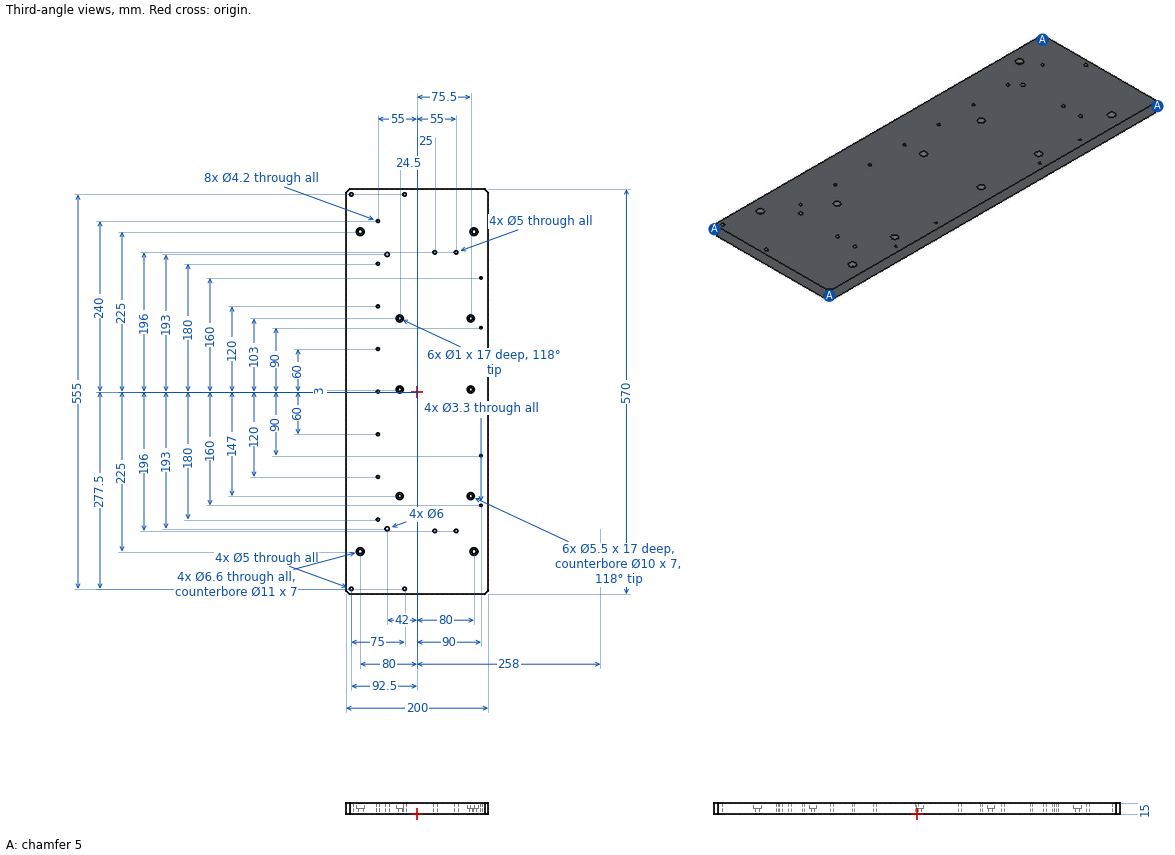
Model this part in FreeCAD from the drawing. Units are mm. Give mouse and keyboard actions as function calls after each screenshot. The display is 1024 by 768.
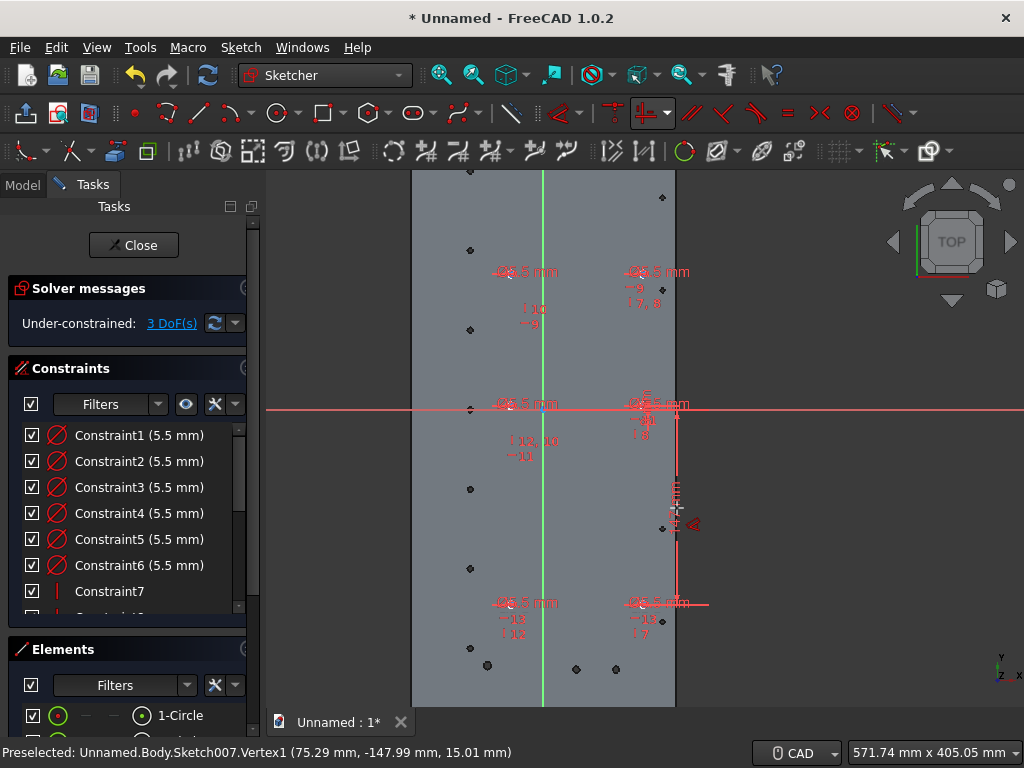
click(643, 274)
click(677, 342)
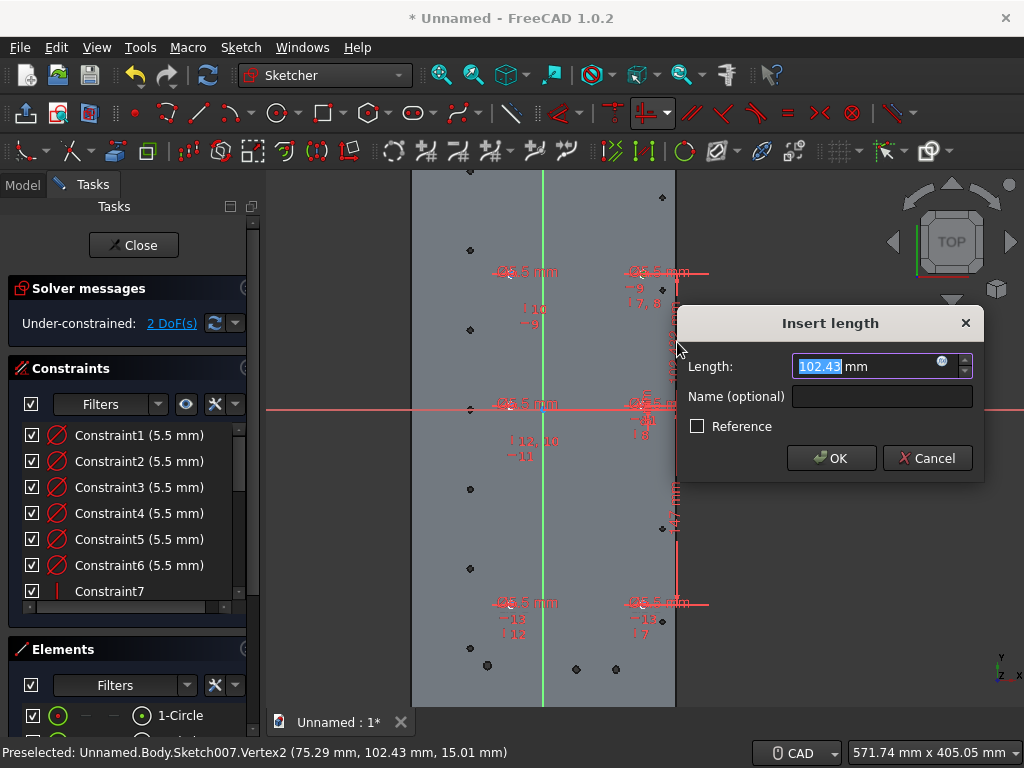
text(103)
key(Return)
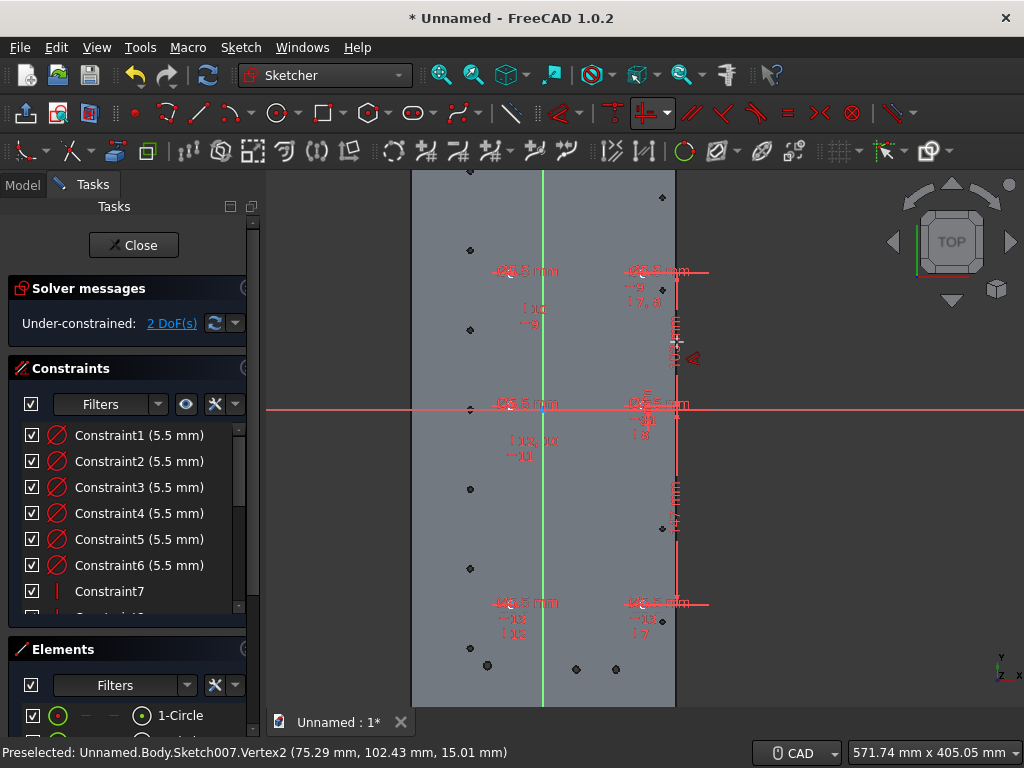
click(643, 605)
click(593, 639)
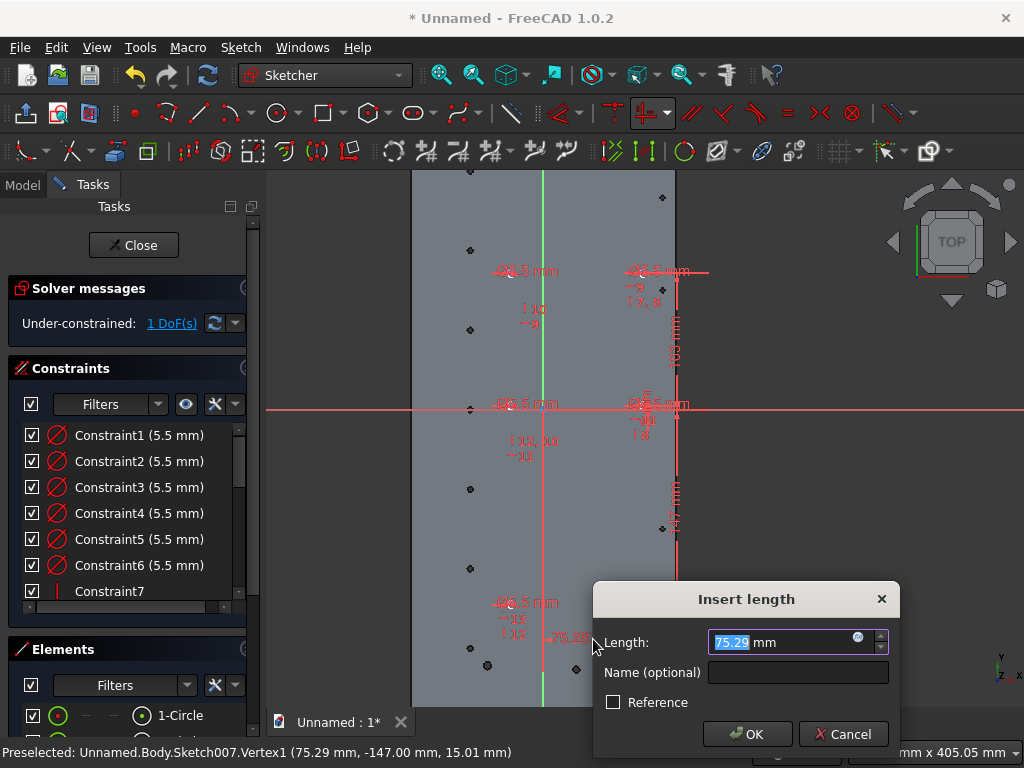
text(75.5)
key(Return)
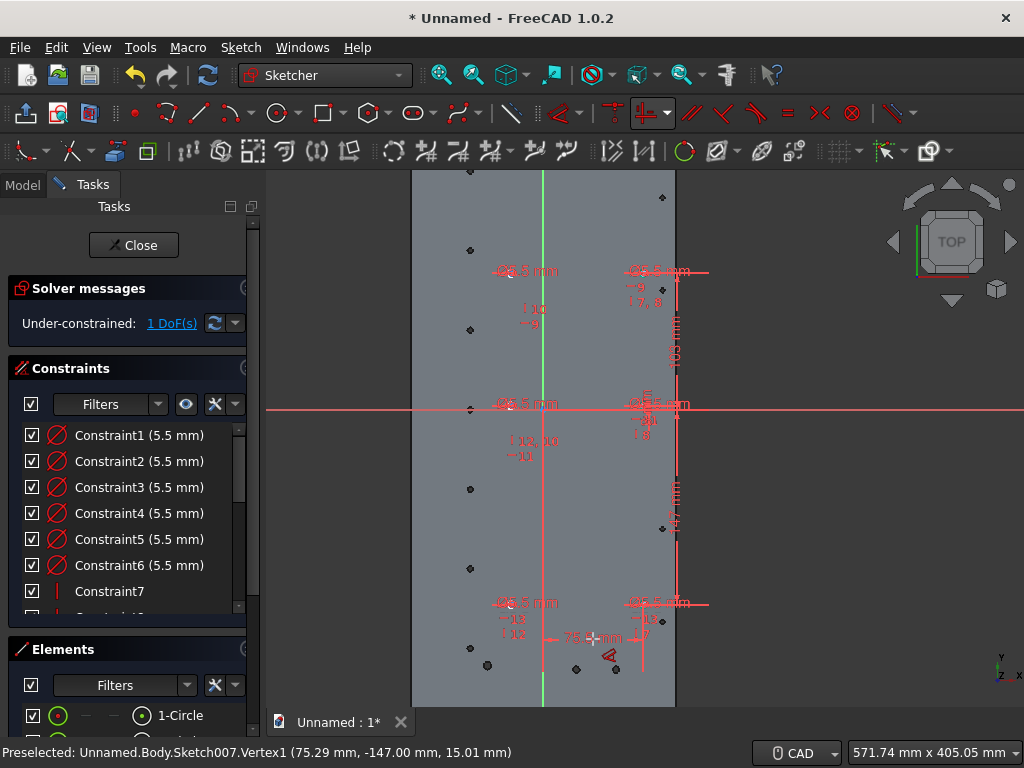
scroll(511, 273, up, 2)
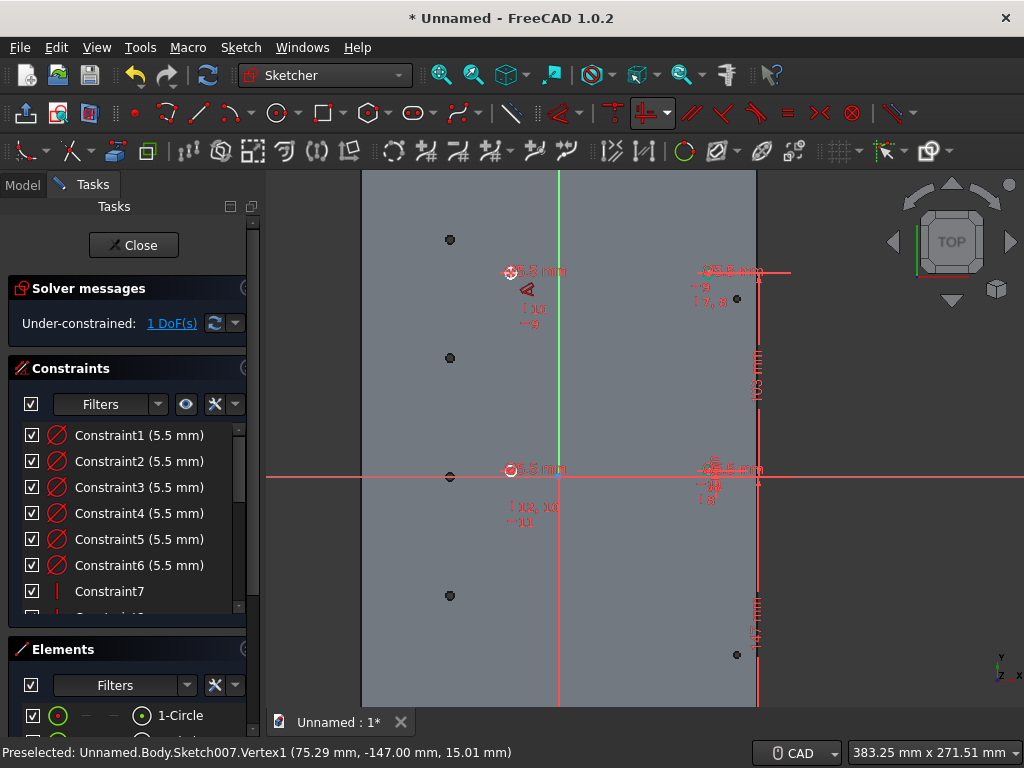
click(511, 273)
click(535, 239)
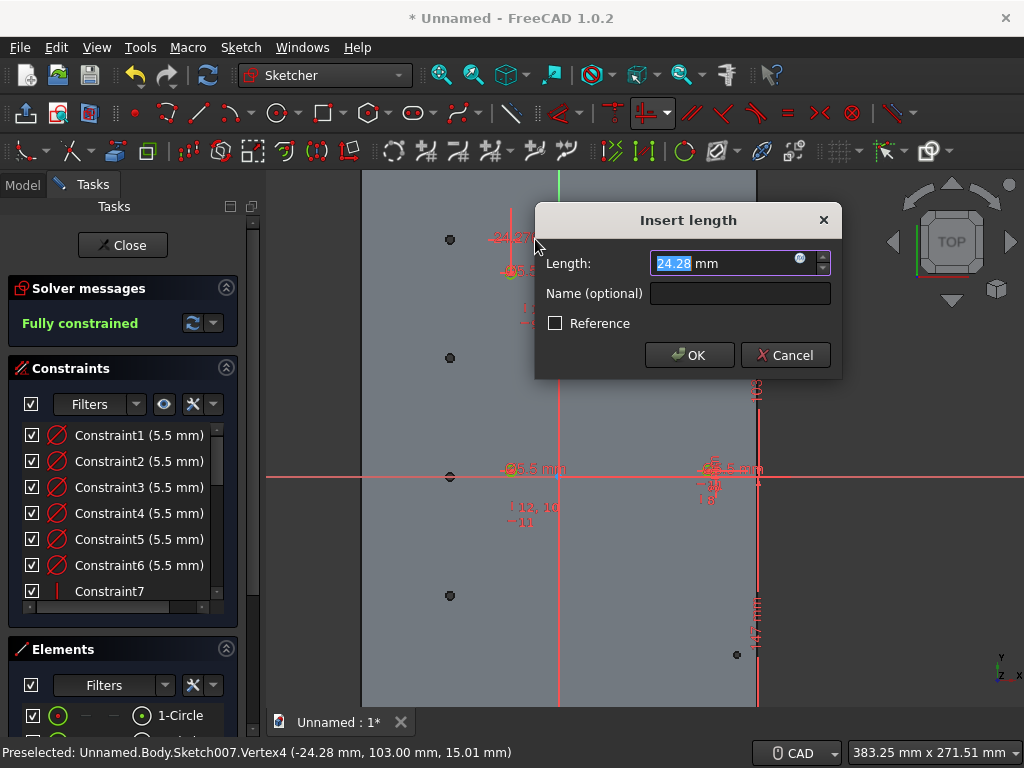
text(24.5)
key(Return)
key(Escape)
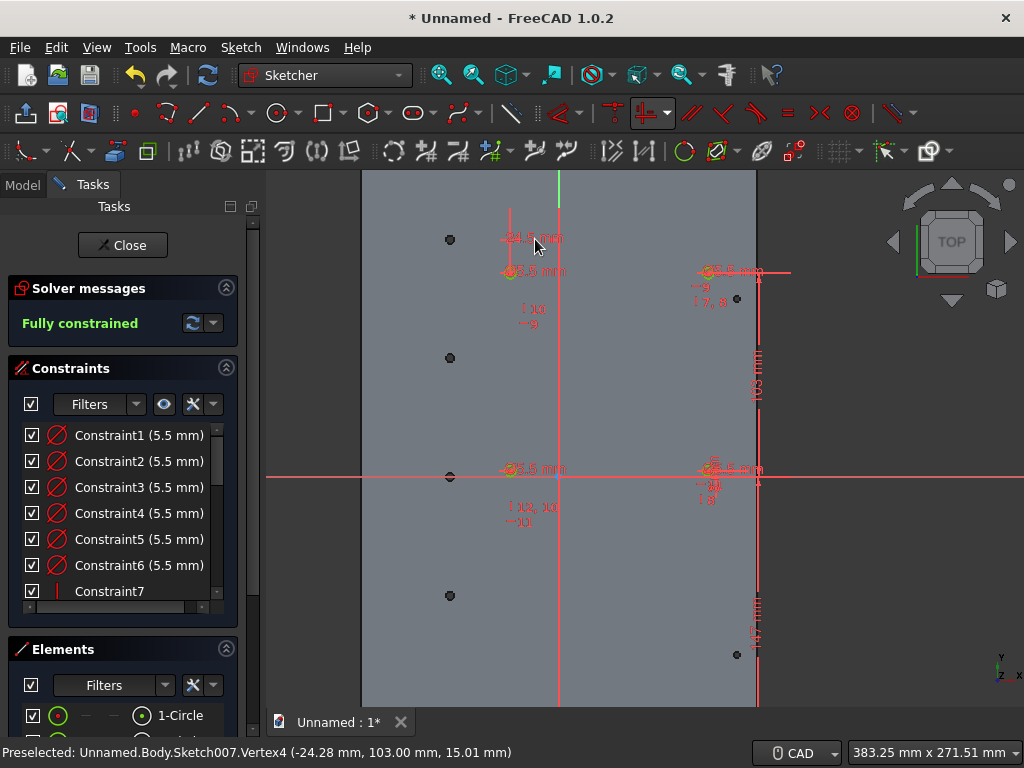
click(123, 245)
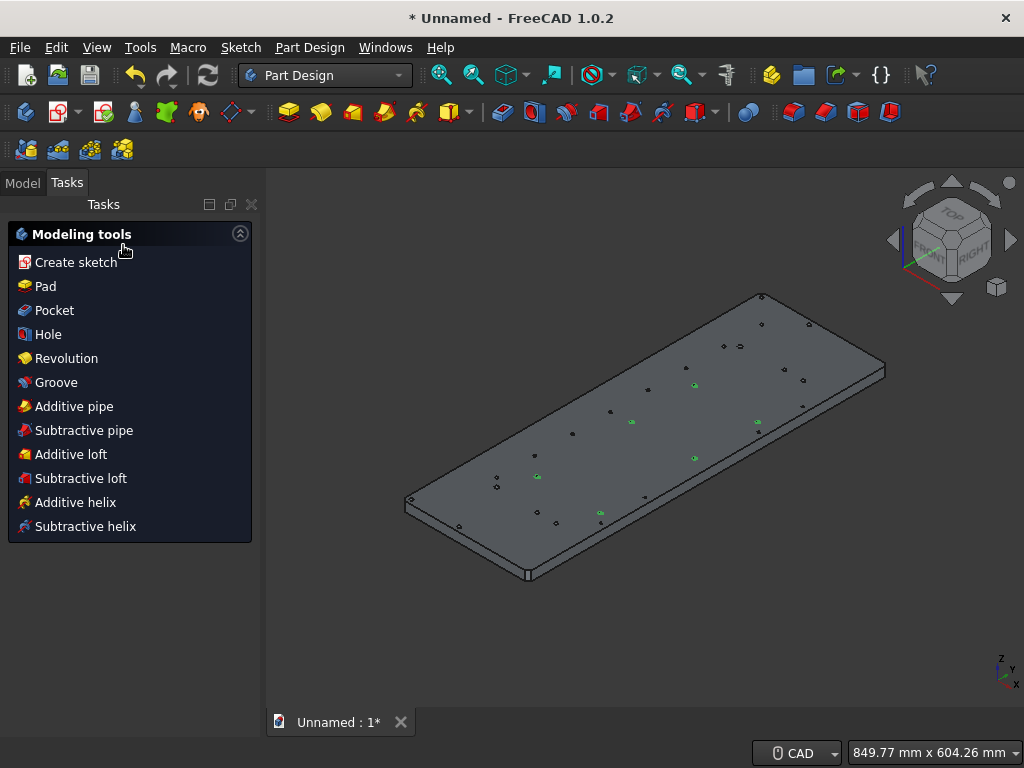
click(536, 112)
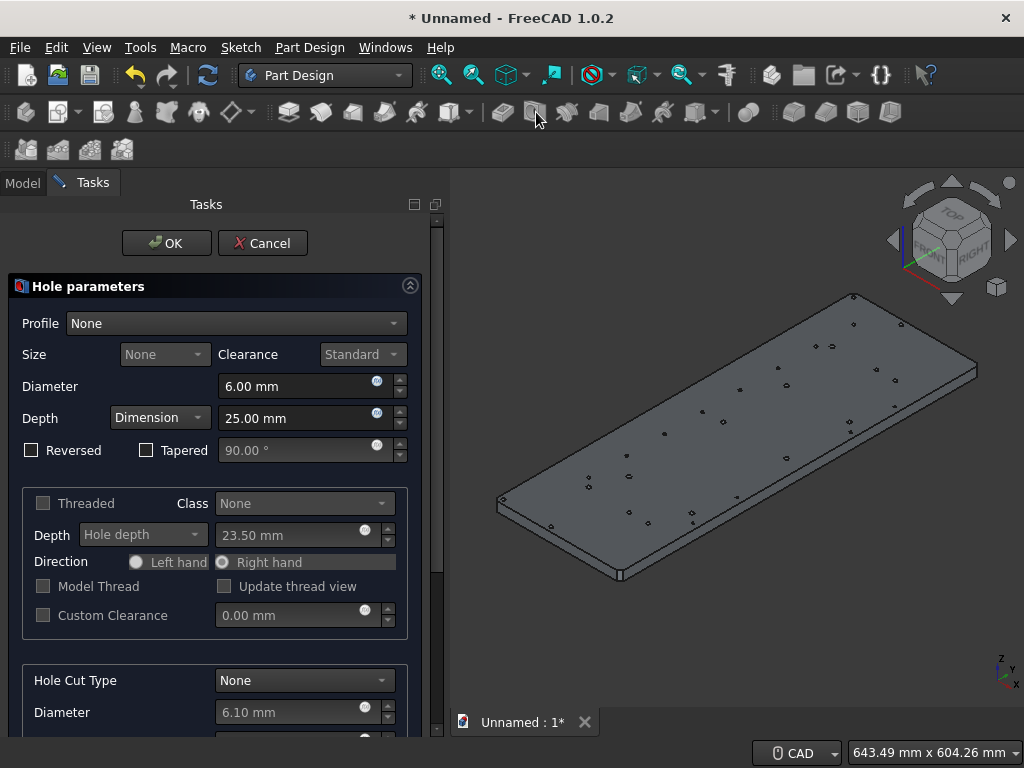
triple_click(305, 386)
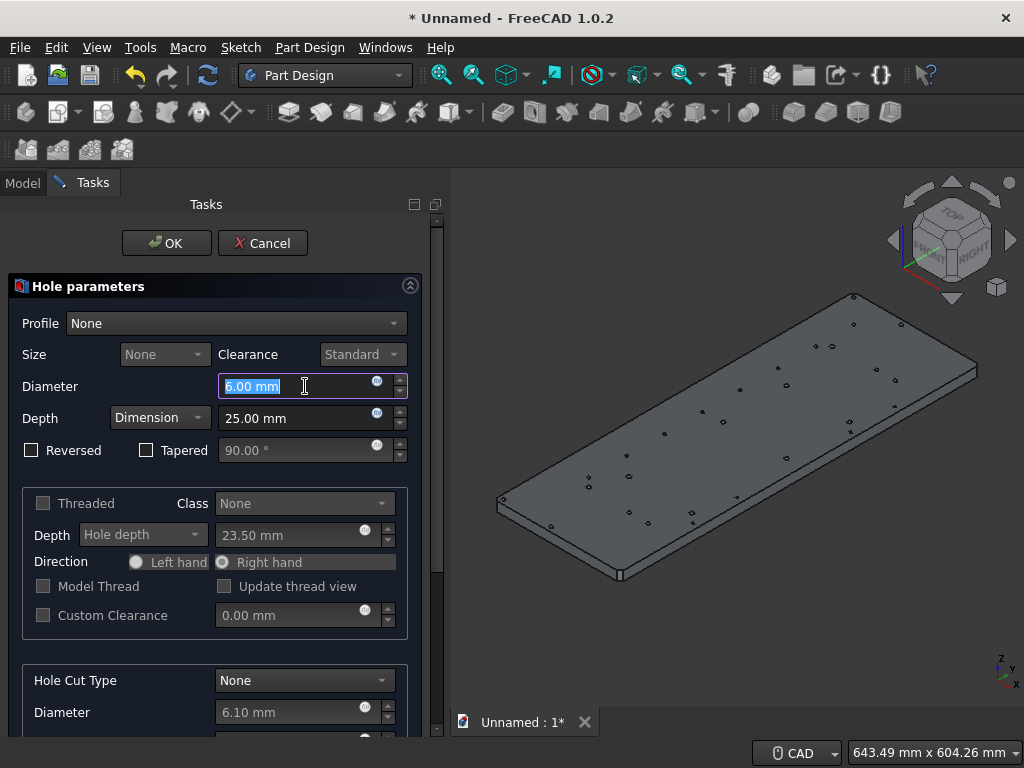
text(5.5)
key(Tab)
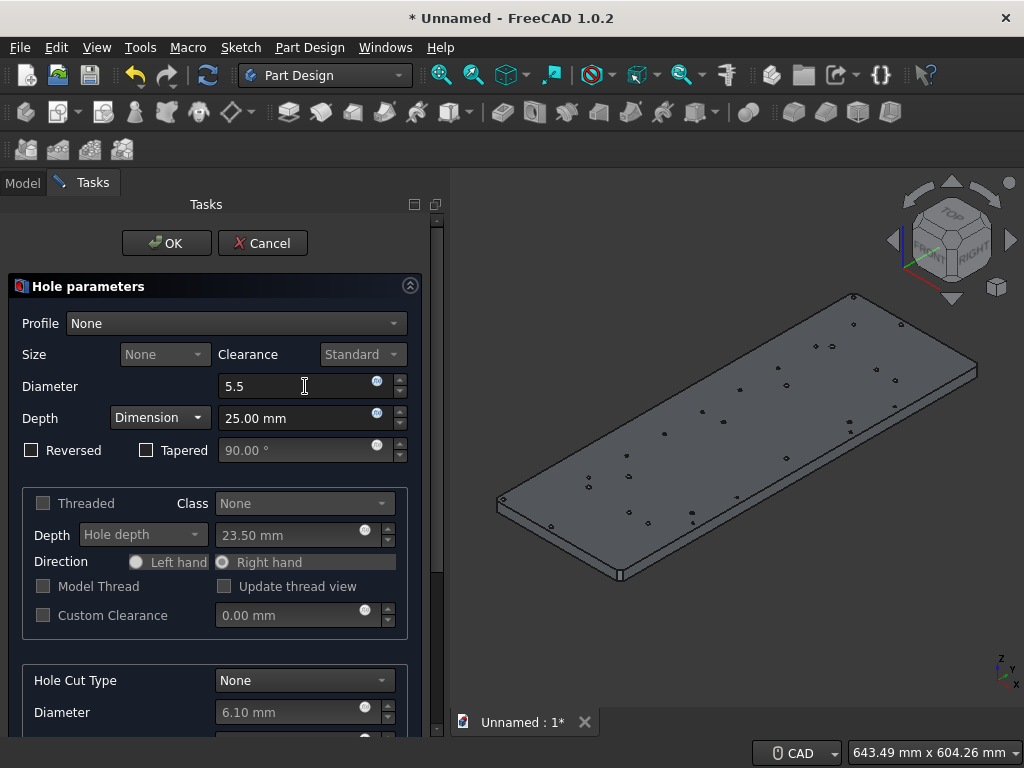
triple_click(305, 418)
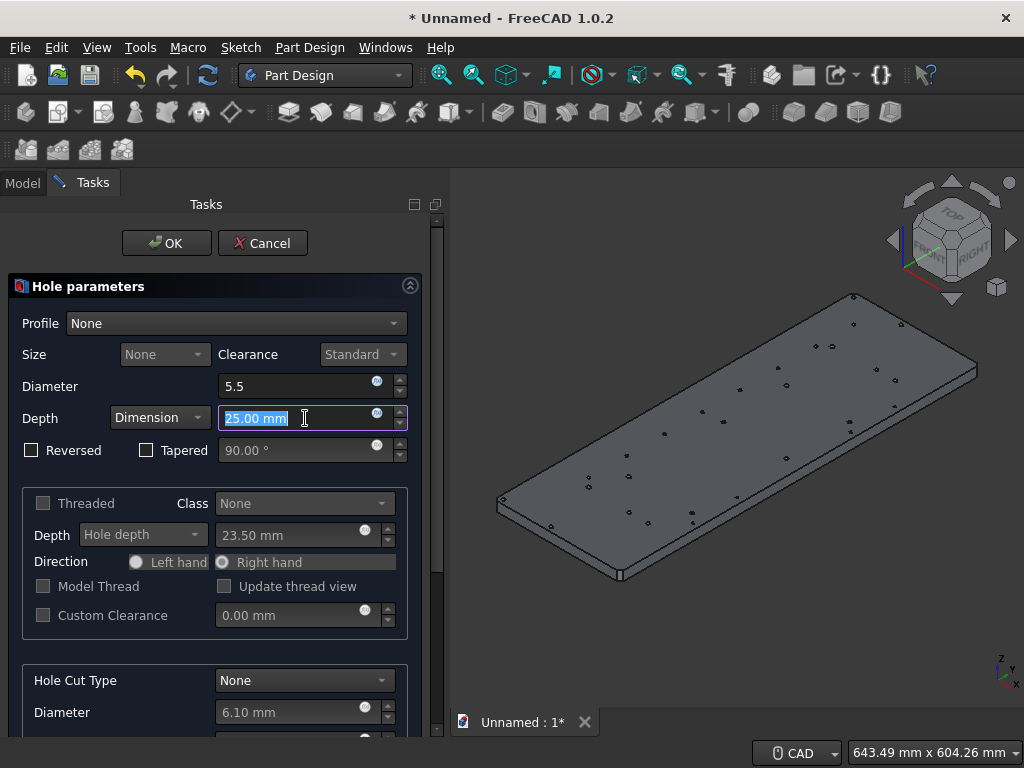
text(17)
key(Tab)